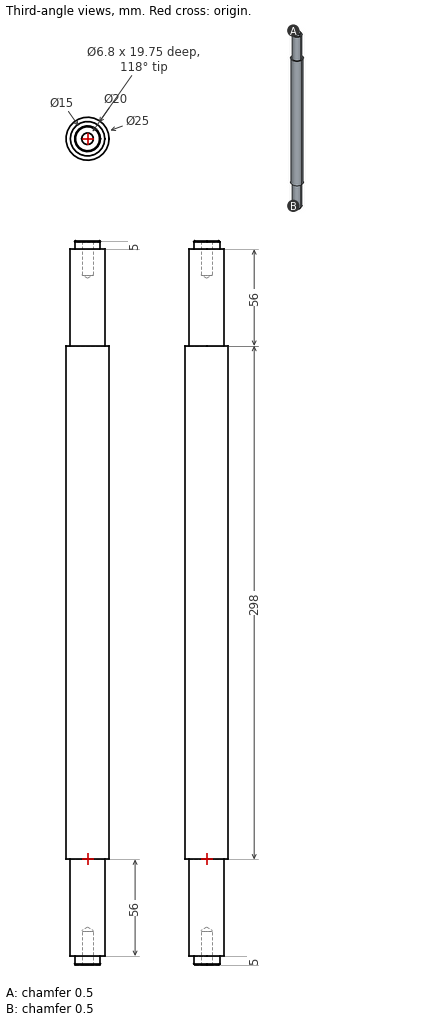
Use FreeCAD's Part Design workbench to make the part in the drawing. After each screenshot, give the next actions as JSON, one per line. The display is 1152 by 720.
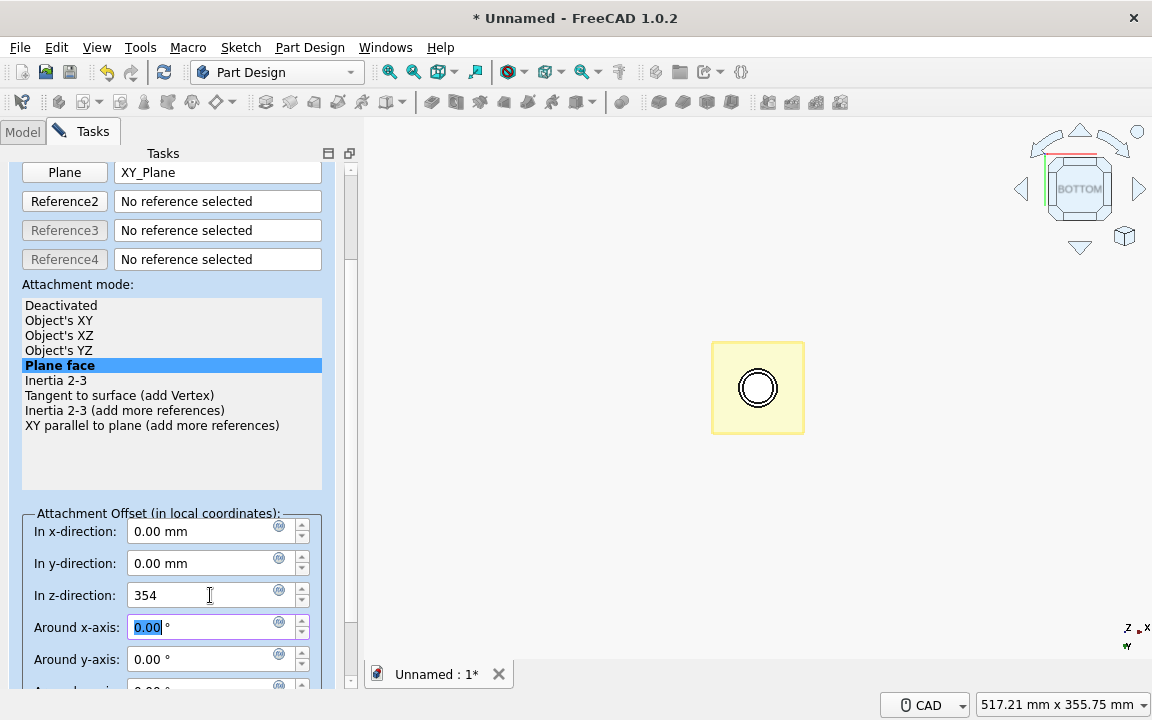
{"action": "scroll", "coordinate": [351, 426], "scroll_direction": "up", "scroll_amount": 3}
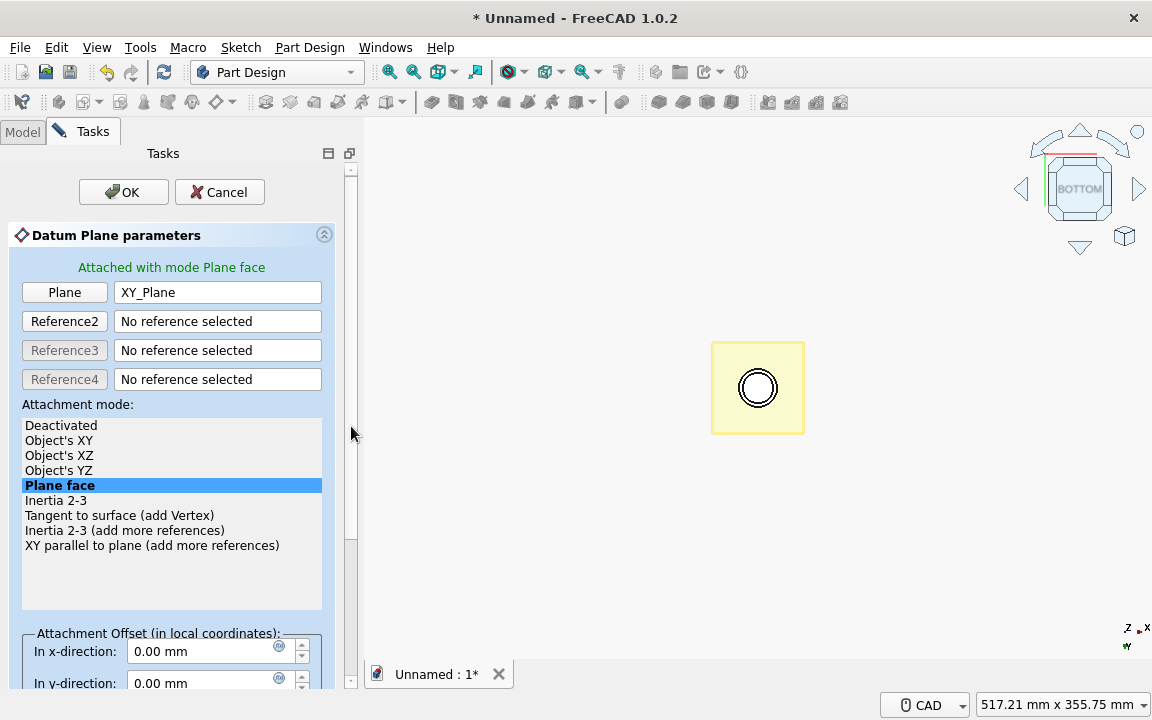
{"action": "left_click", "coordinate": [124, 192]}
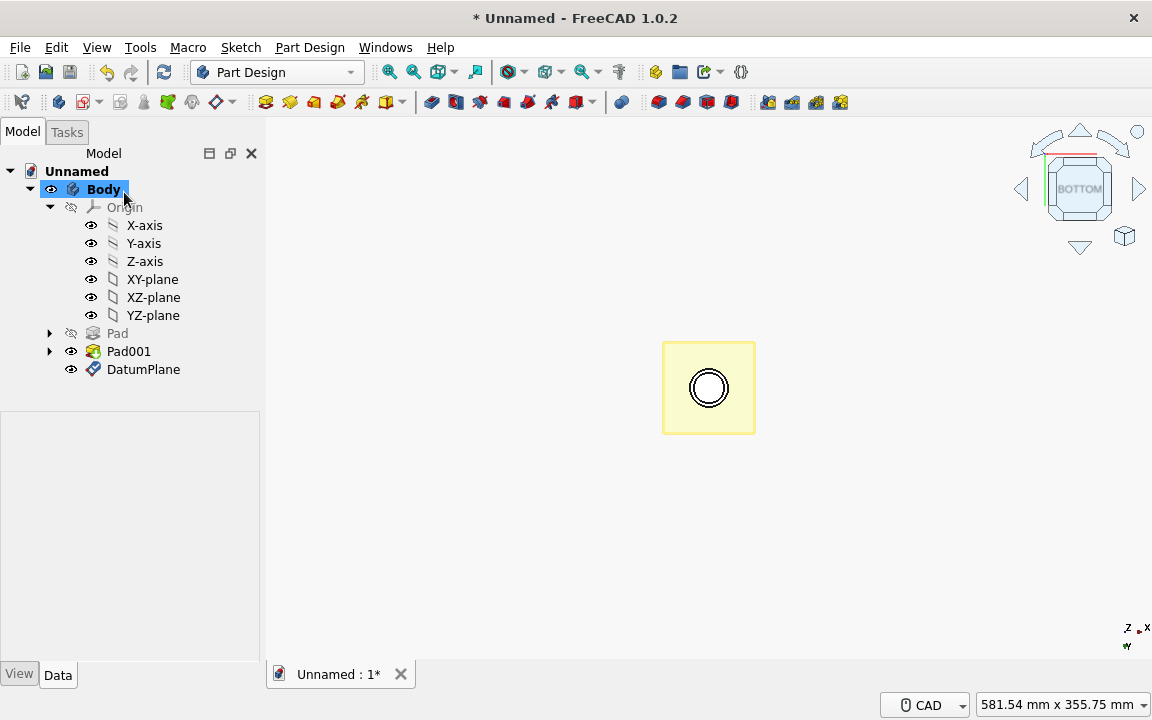
{"action": "left_click", "coordinate": [116, 369]}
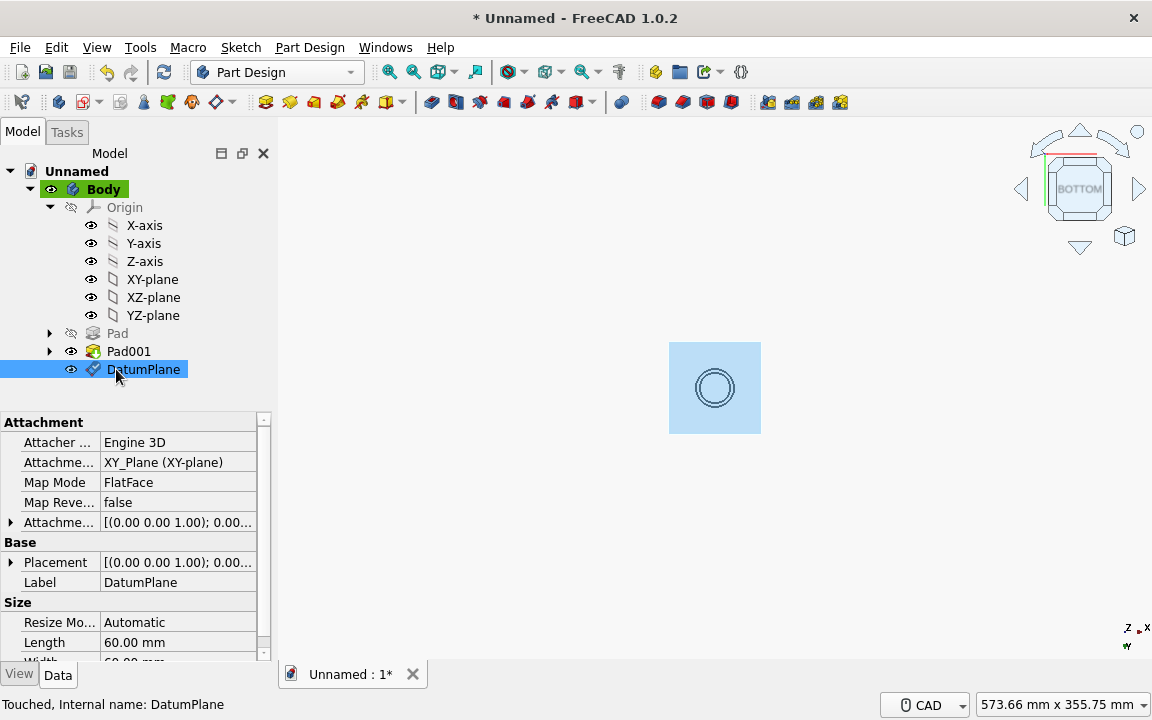
{"action": "left_click", "coordinate": [84, 102]}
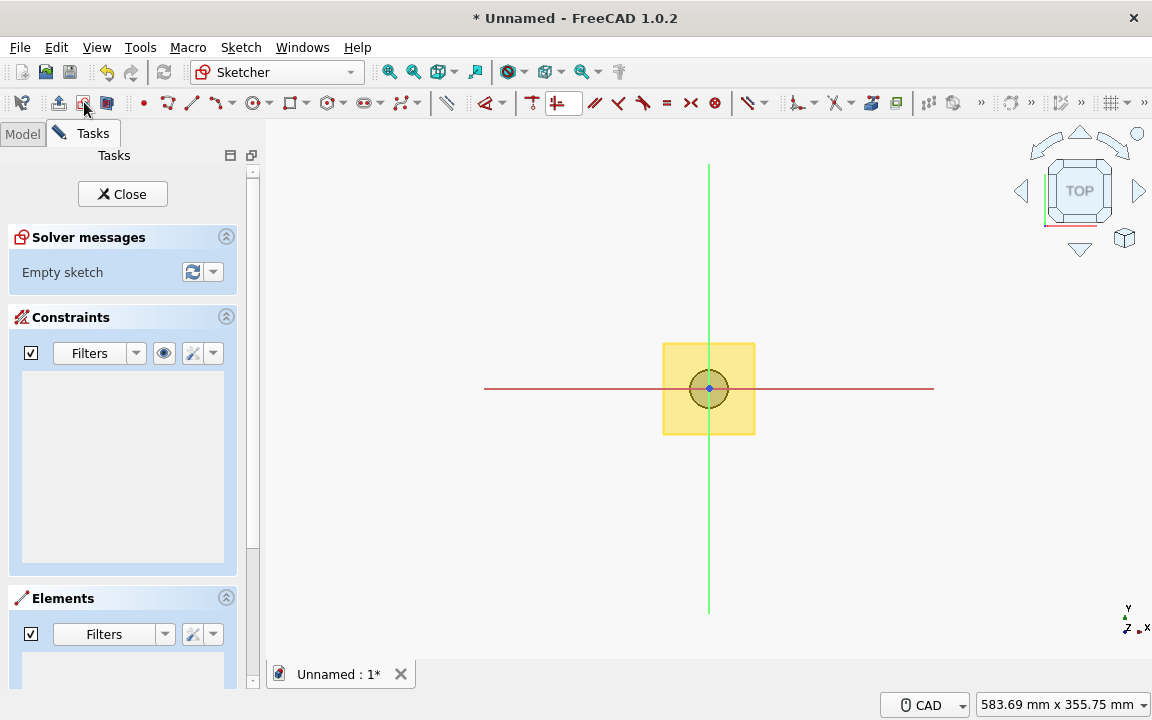
{"action": "scroll", "coordinate": [716, 389], "scroll_direction": "up", "scroll_amount": 12}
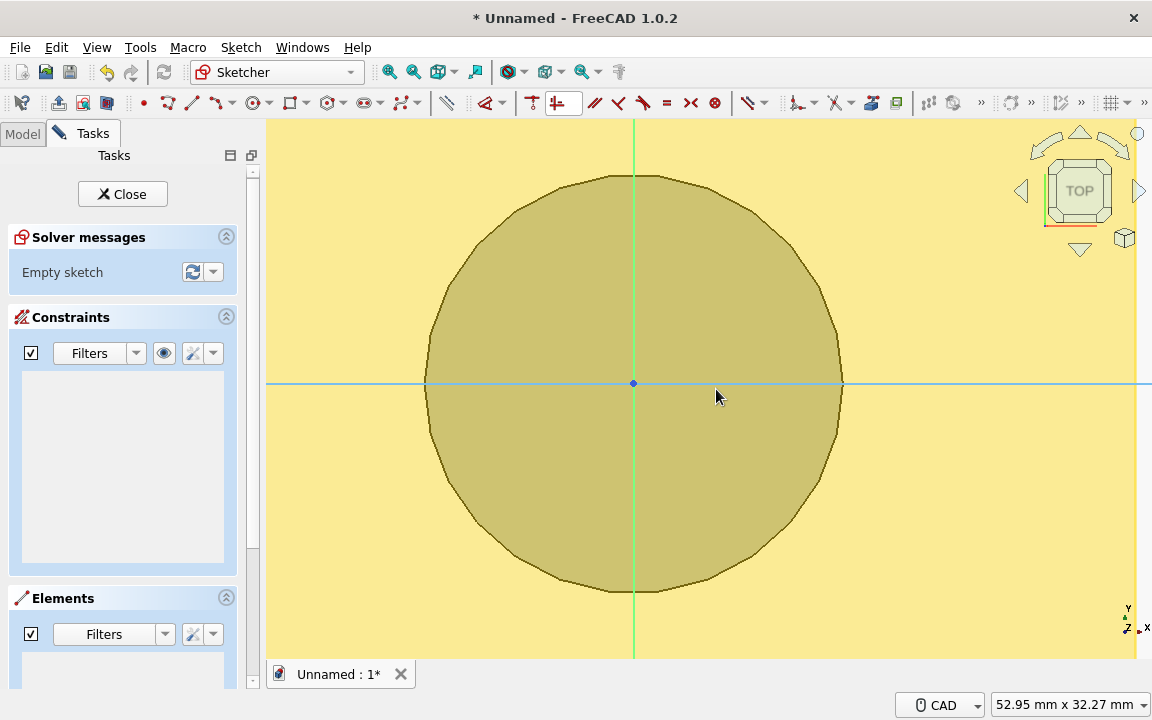
{"action": "left_click", "coordinate": [254, 104]}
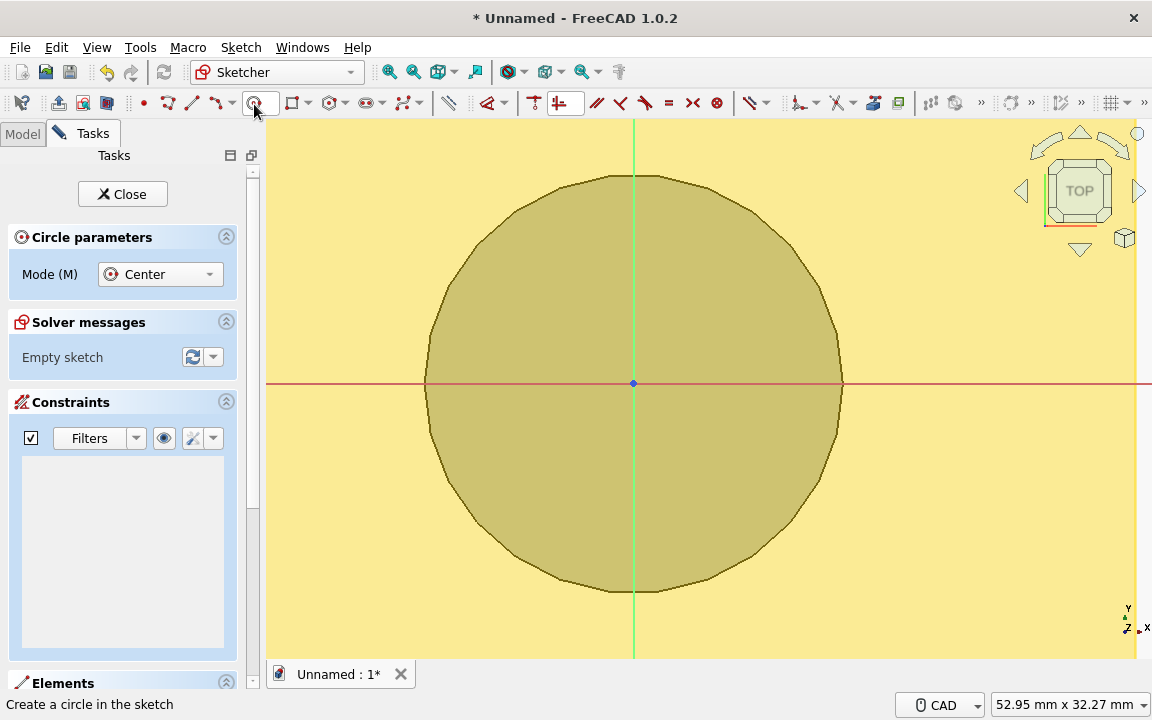
{"action": "left_click", "coordinate": [634, 384]}
{"action": "left_click", "coordinate": [752, 266]}
{"action": "key", "text": "Escape"}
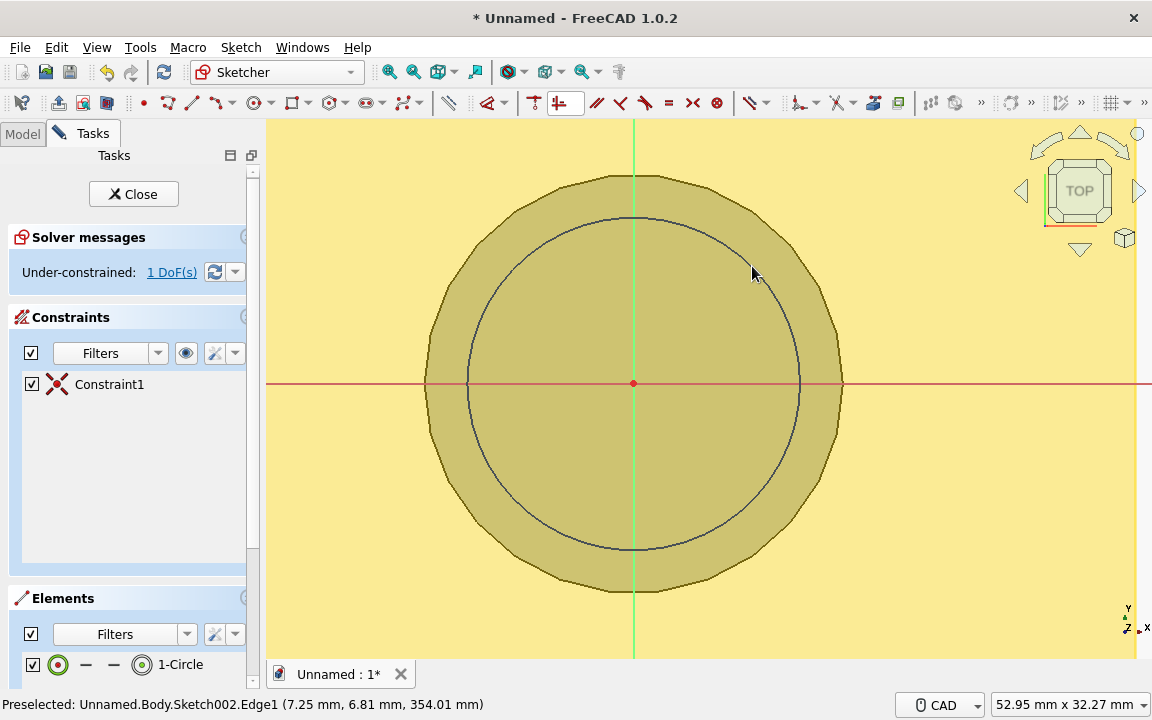
{"action": "left_click", "coordinate": [488, 104]}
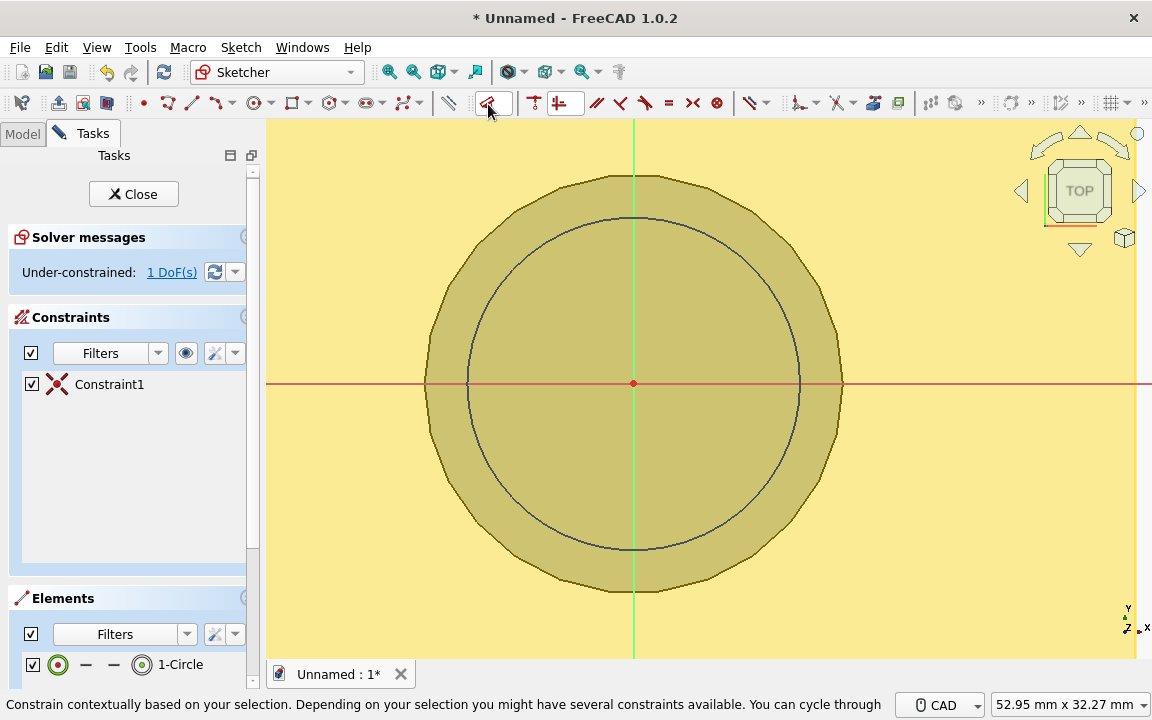
{"action": "left_click", "coordinate": [751, 266]}
{"action": "left_click", "coordinate": [774, 243]}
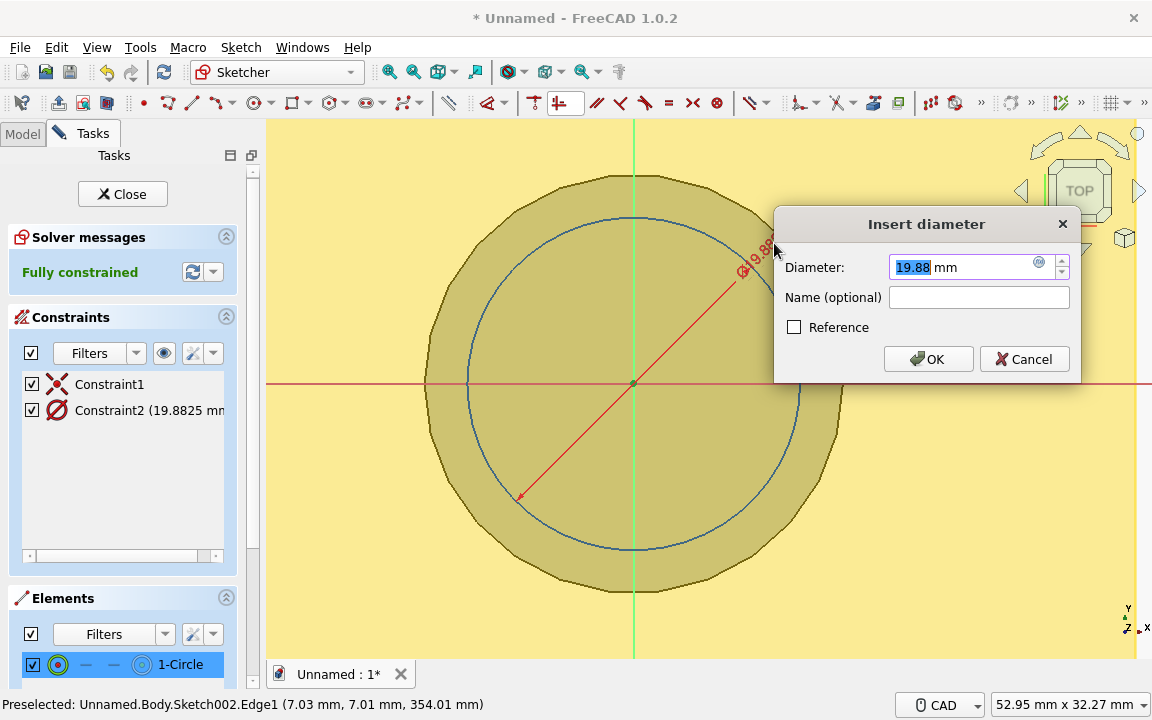
{"action": "type", "text": "20"}
{"action": "key", "text": "Return"}
{"action": "key", "text": "Escape"}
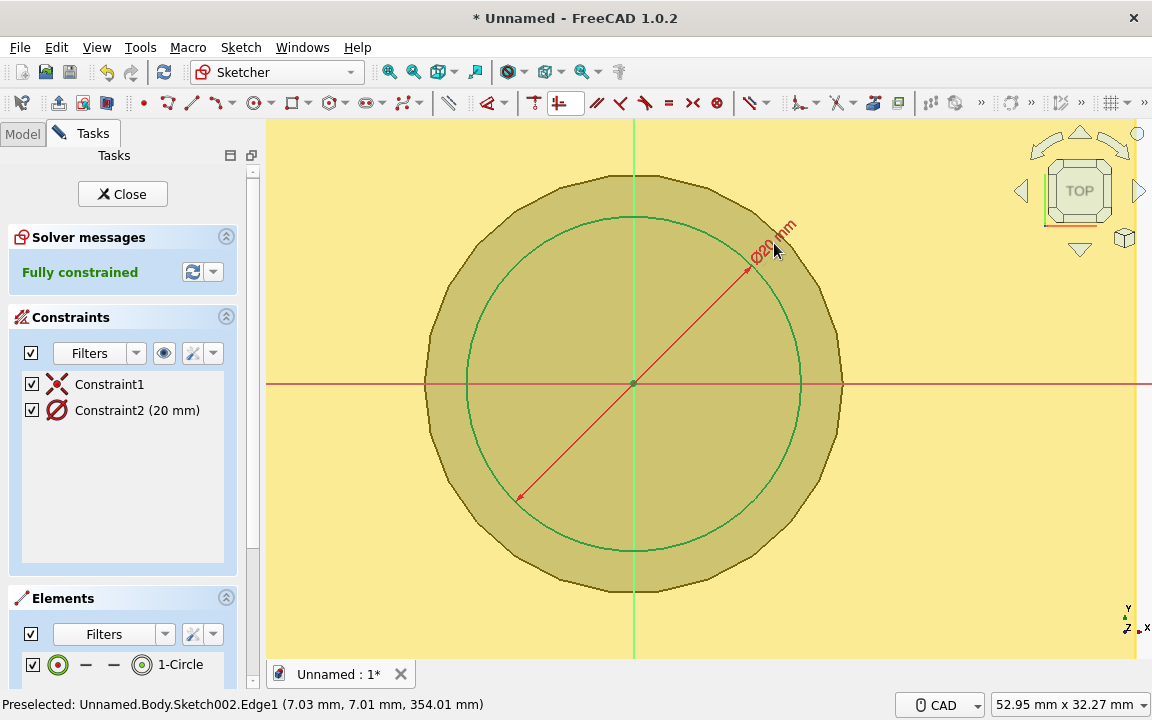
{"action": "left_click", "coordinate": [123, 194]}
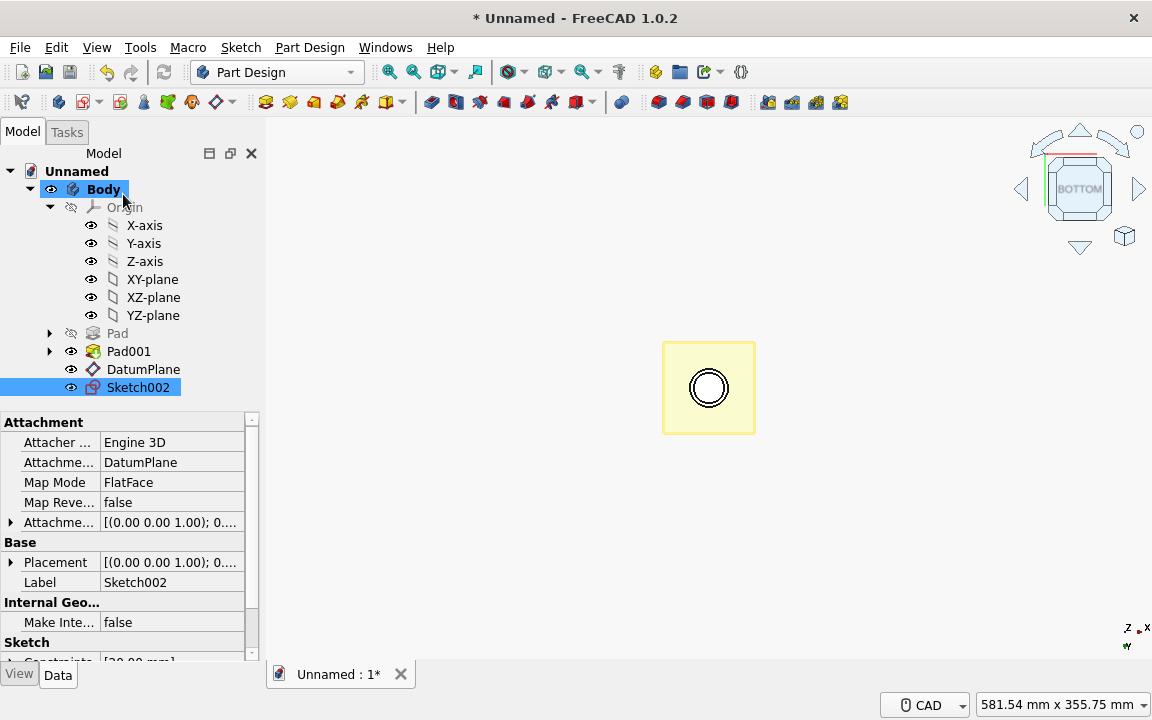
{"action": "left_click", "coordinate": [266, 102]}